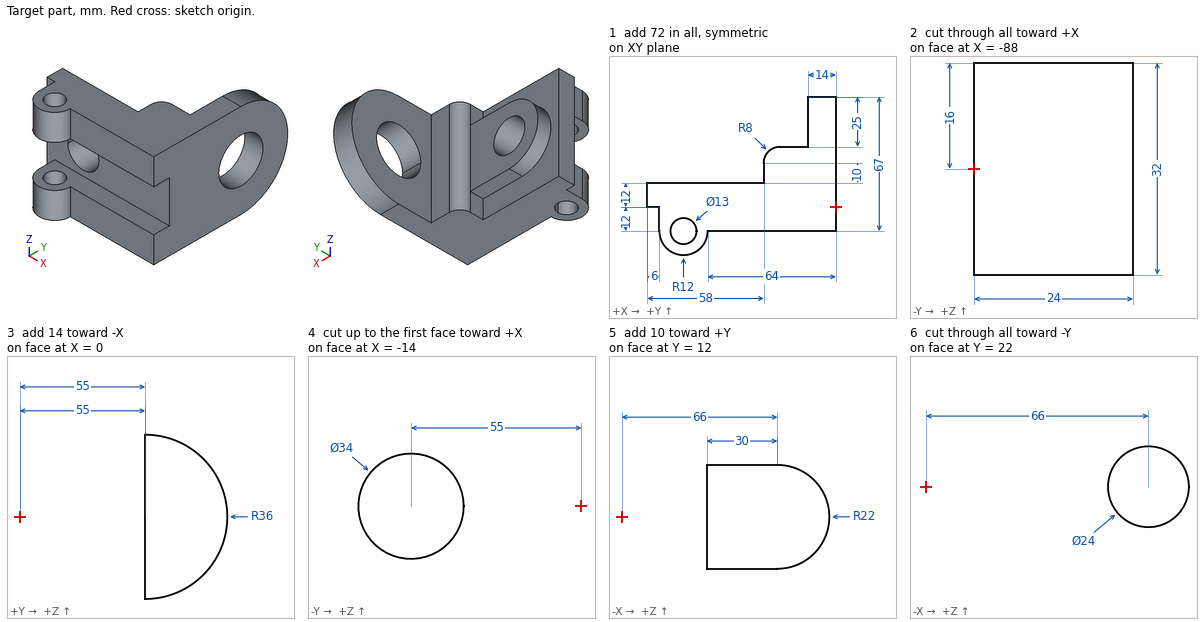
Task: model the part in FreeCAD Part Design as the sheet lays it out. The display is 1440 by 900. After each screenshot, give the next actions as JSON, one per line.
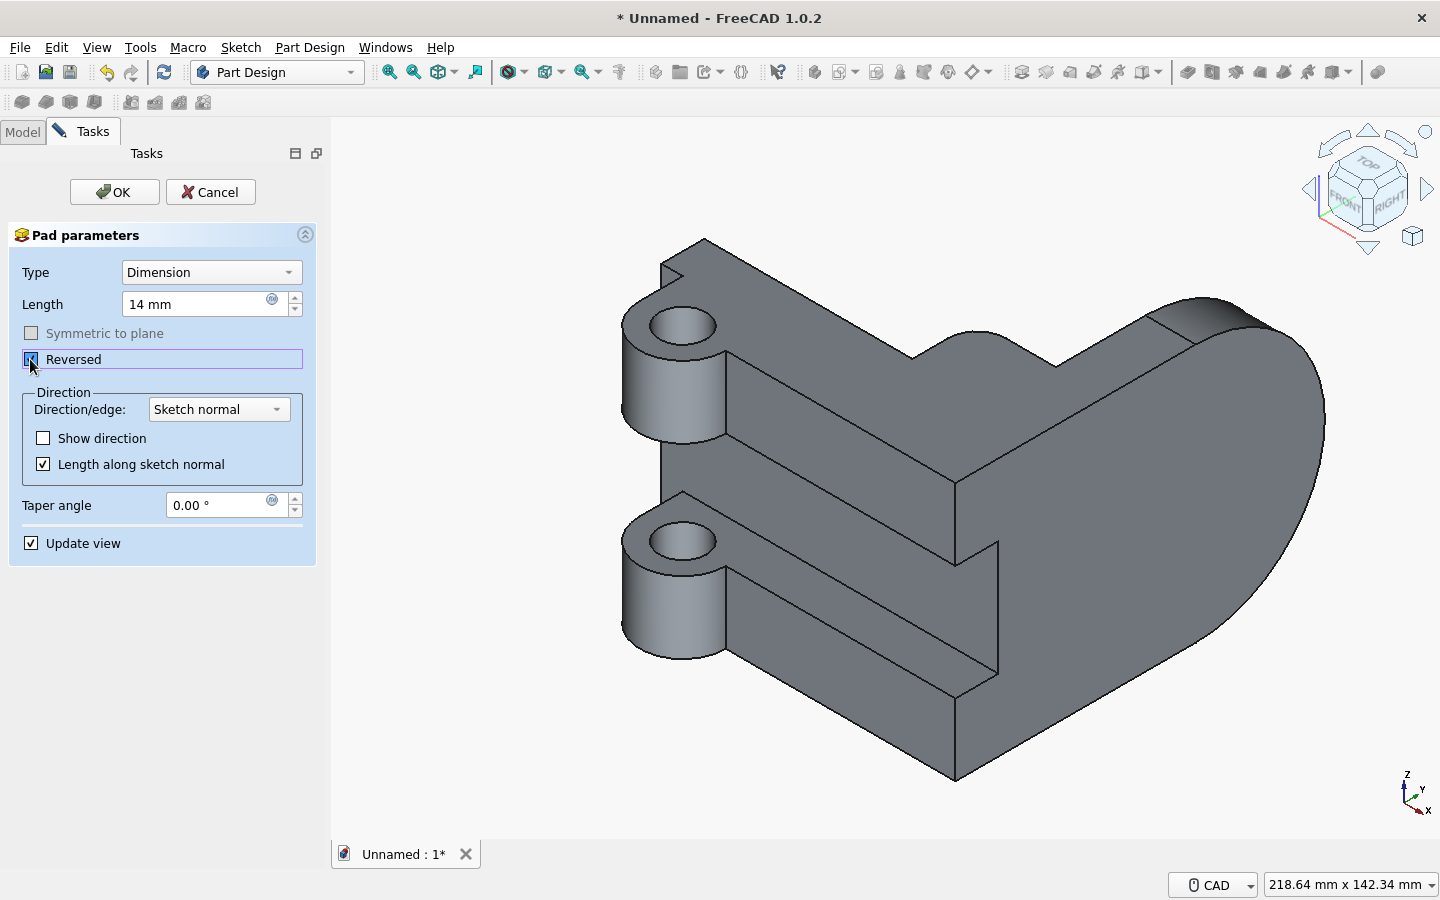
{"action": "left_click", "coordinate": [115, 192]}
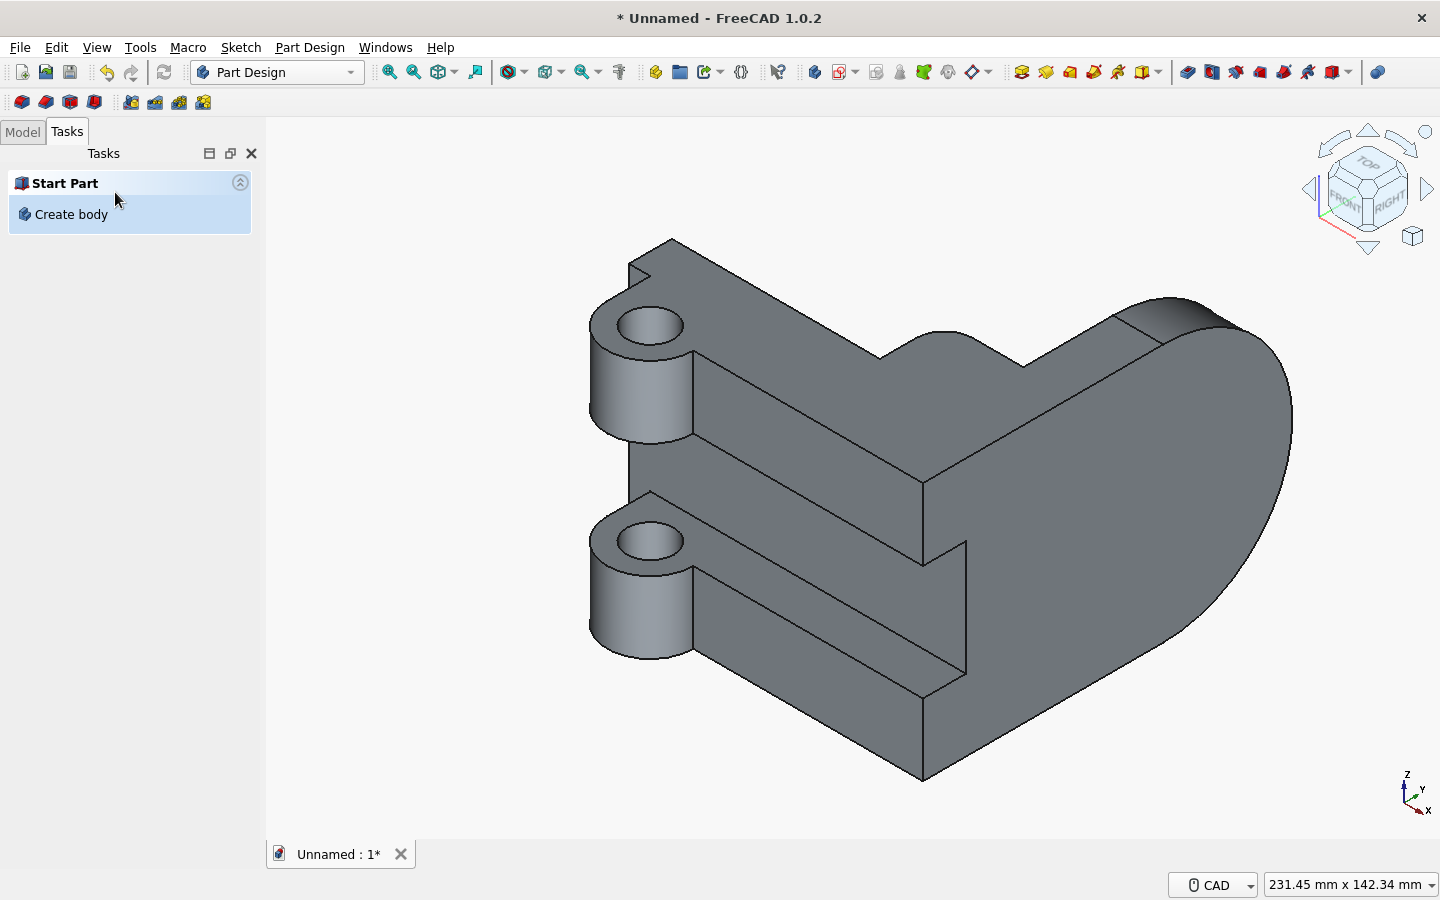
{"action": "left_click", "coordinate": [390, 72]}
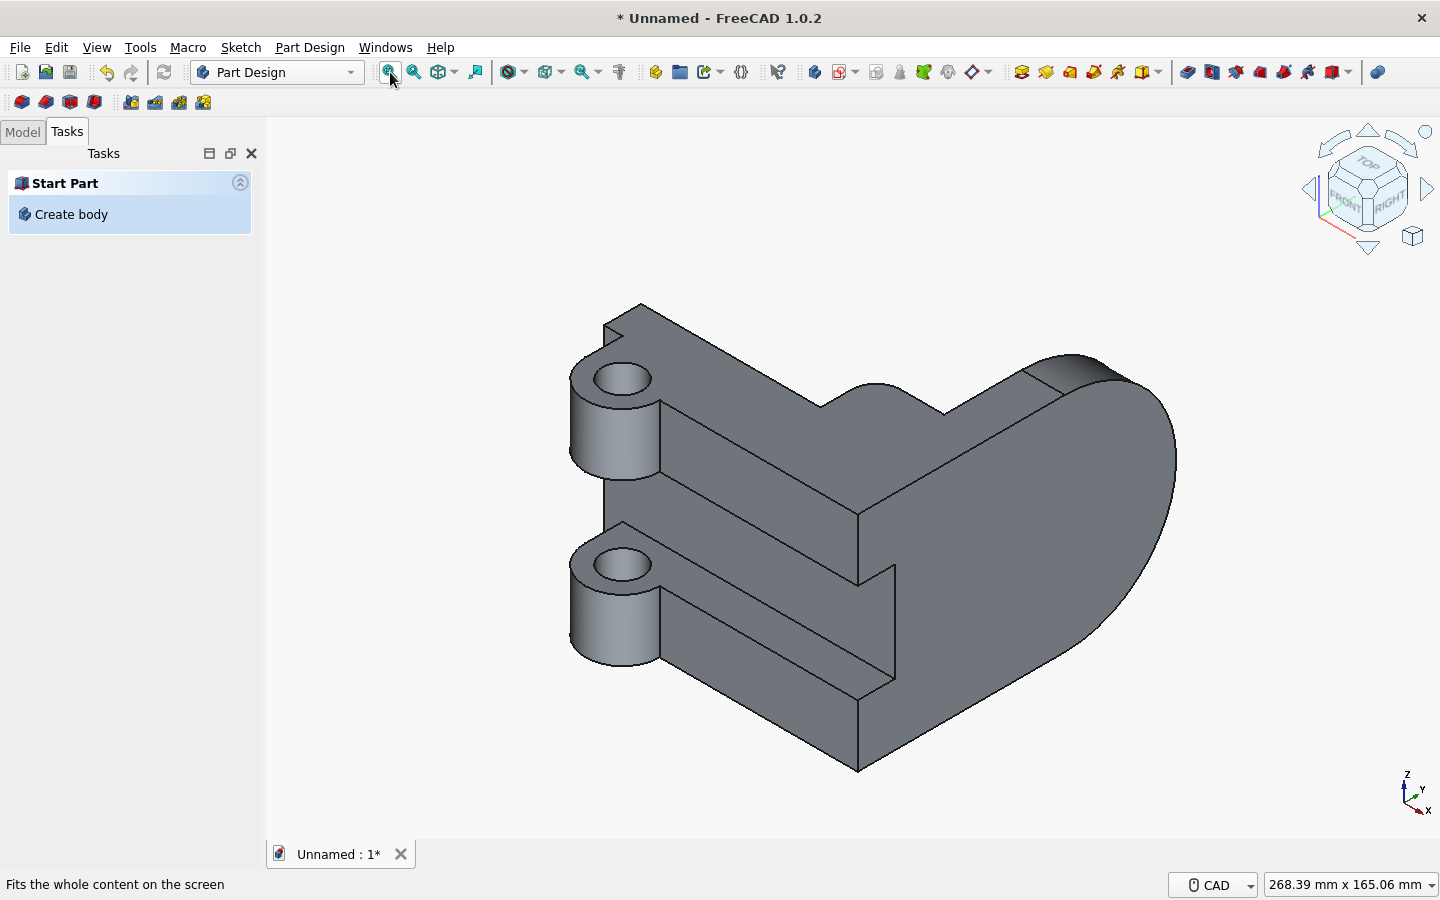
{"action": "key", "text": "6"}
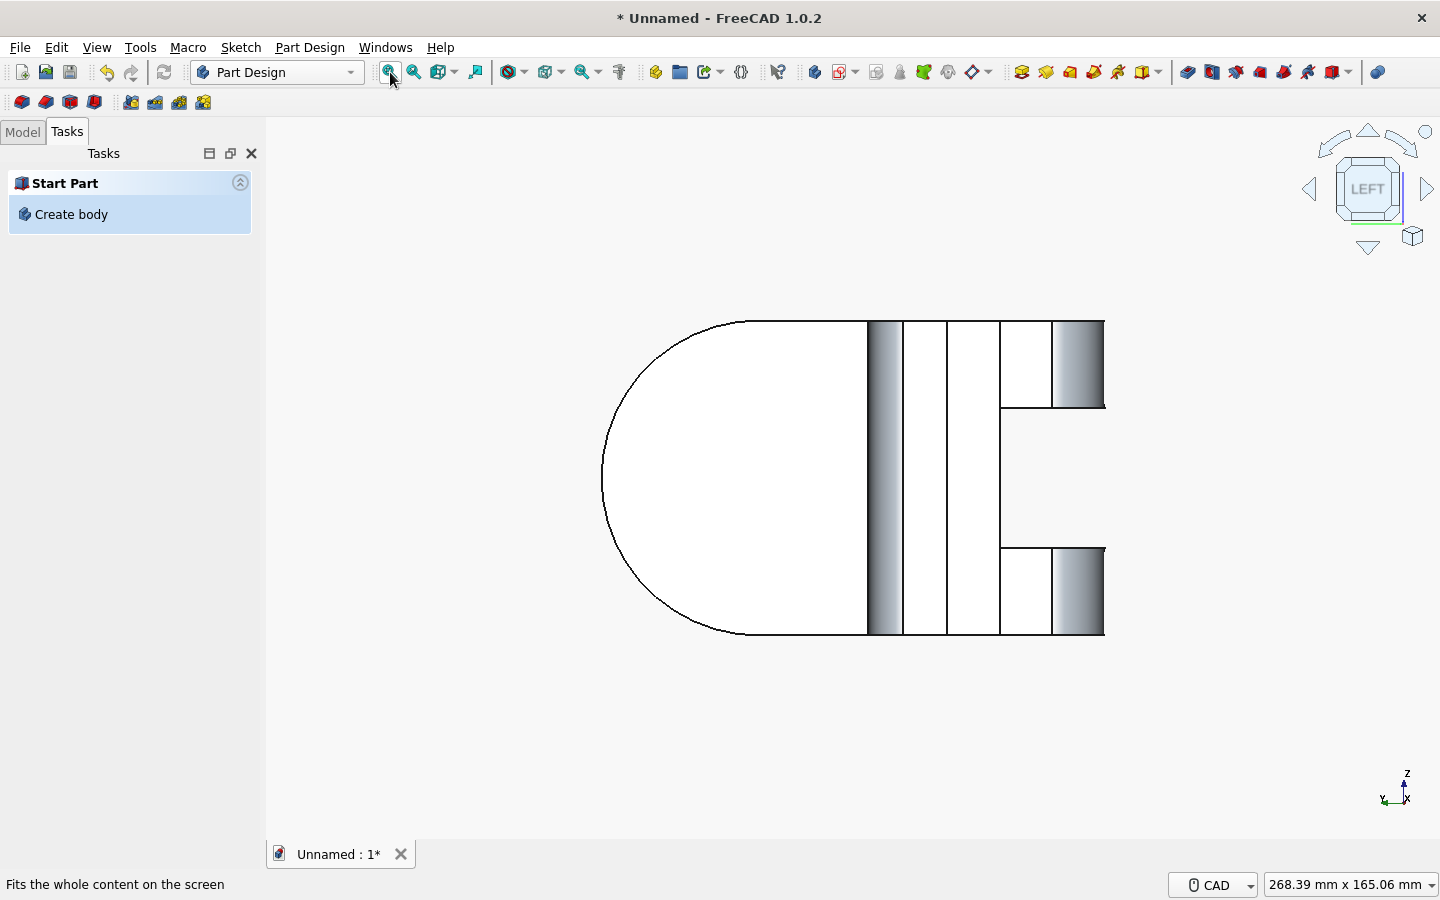
{"action": "left_click", "coordinate": [390, 72]}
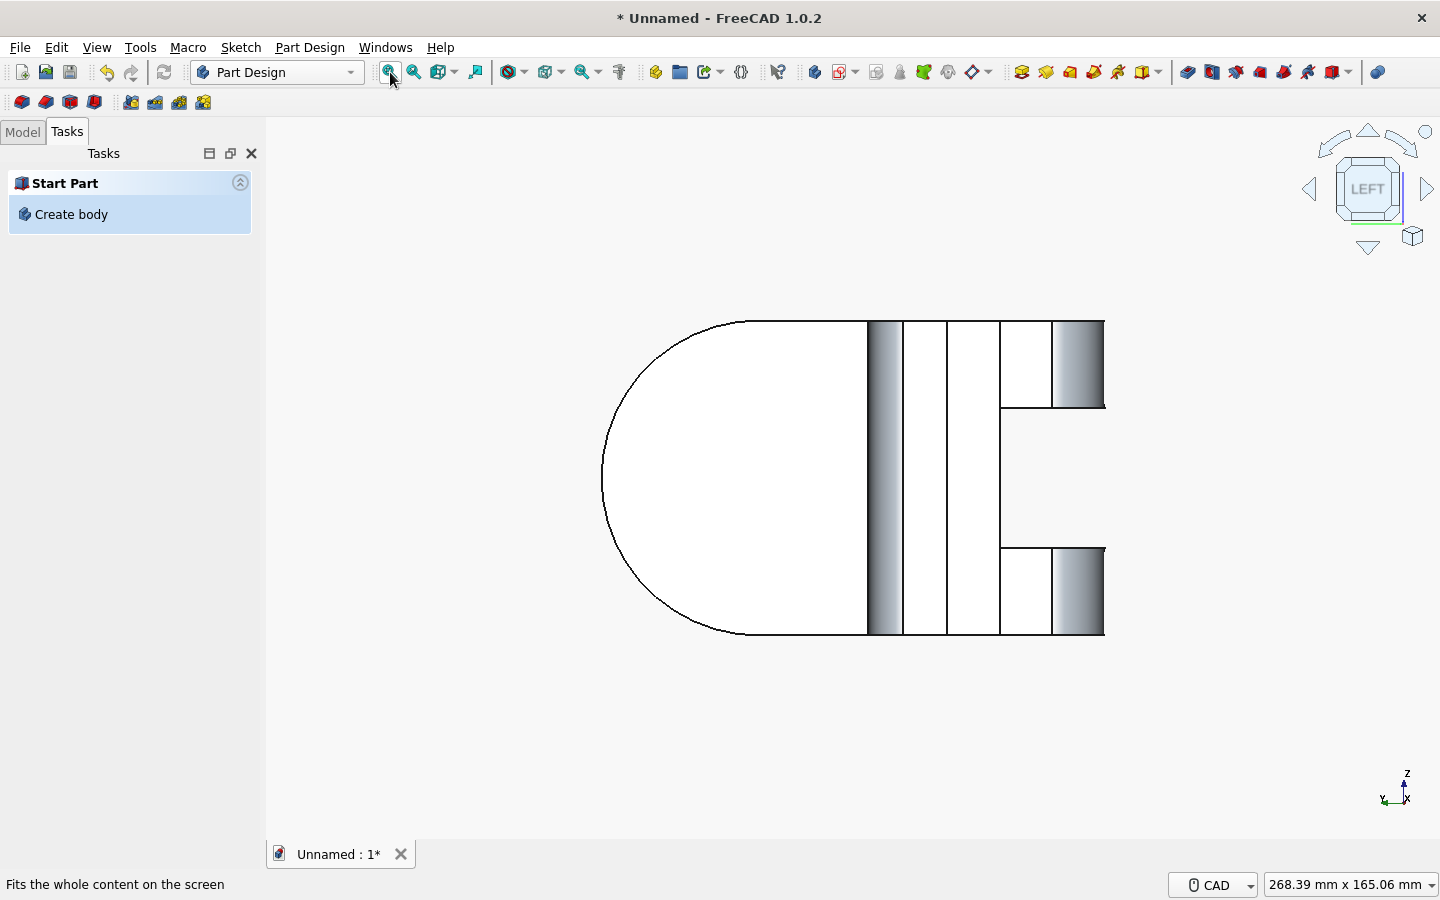
{"action": "left_click", "coordinate": [735, 477]}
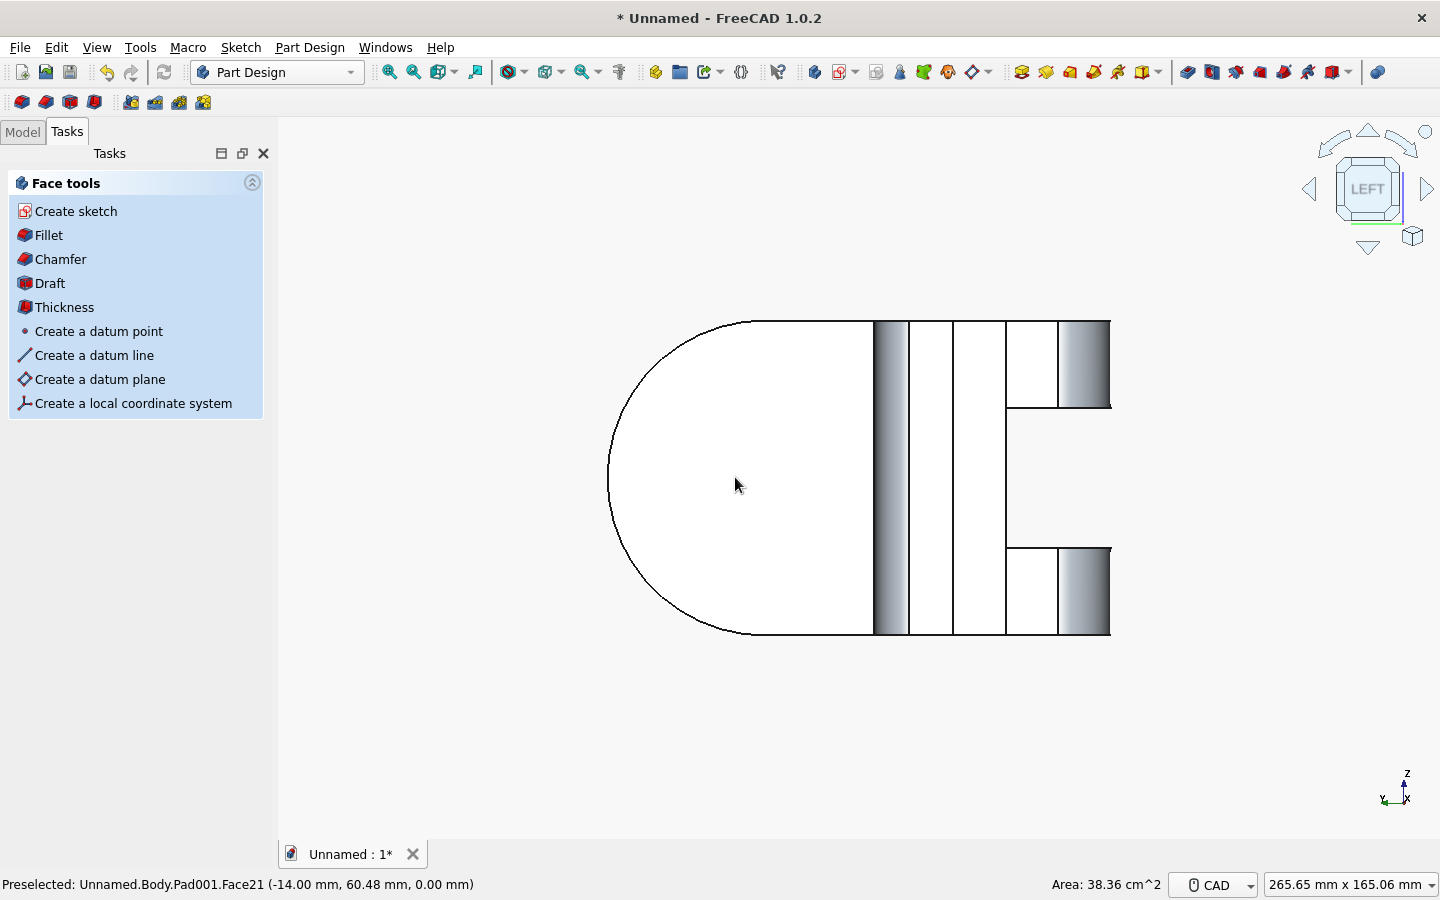
{"action": "left_click", "coordinate": [840, 72]}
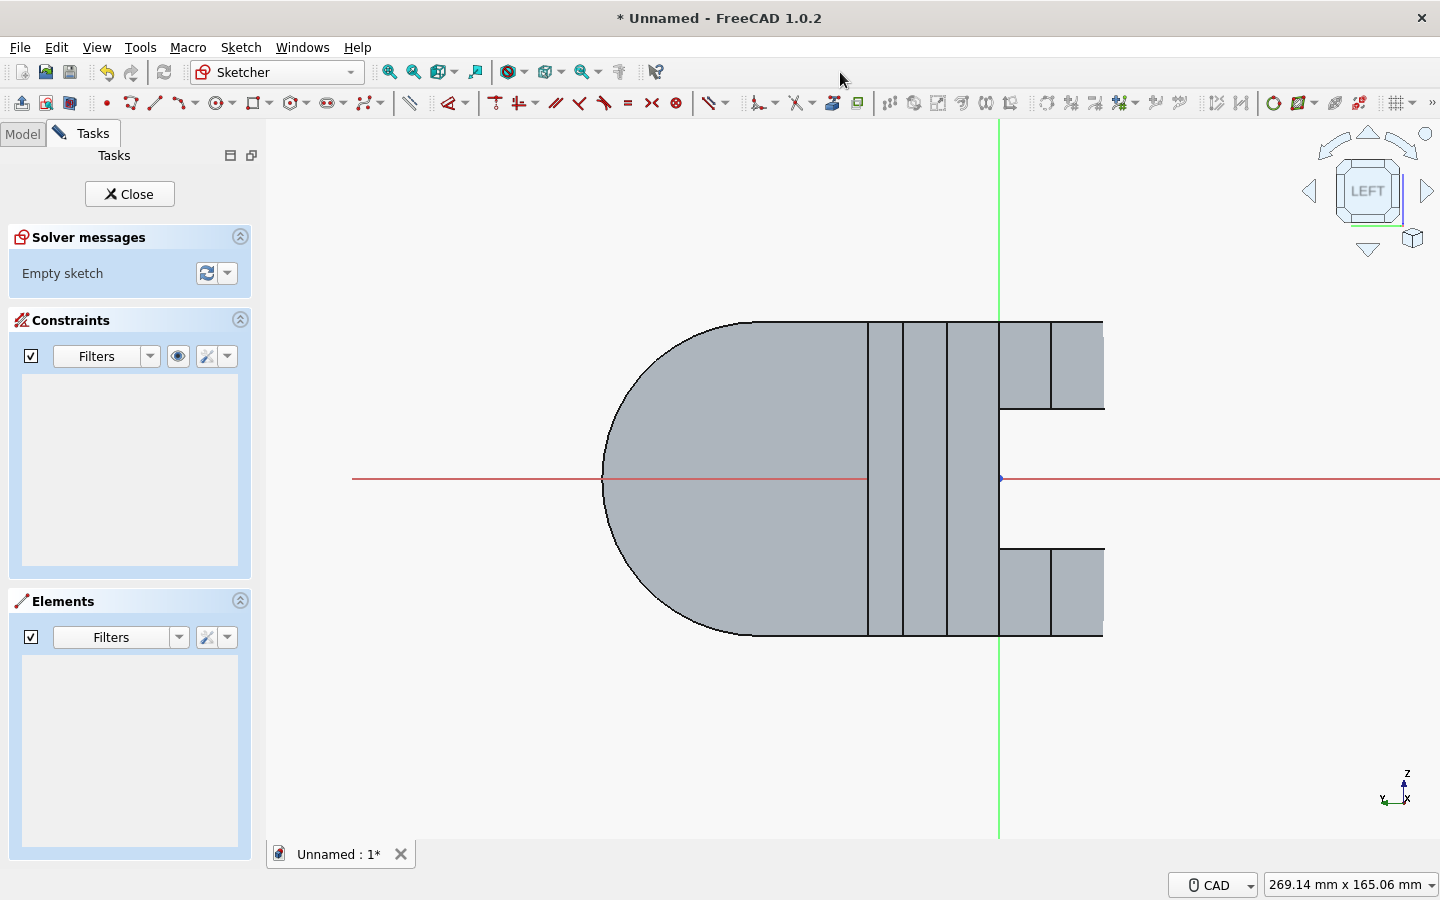
{"action": "left_click", "coordinate": [70, 104]}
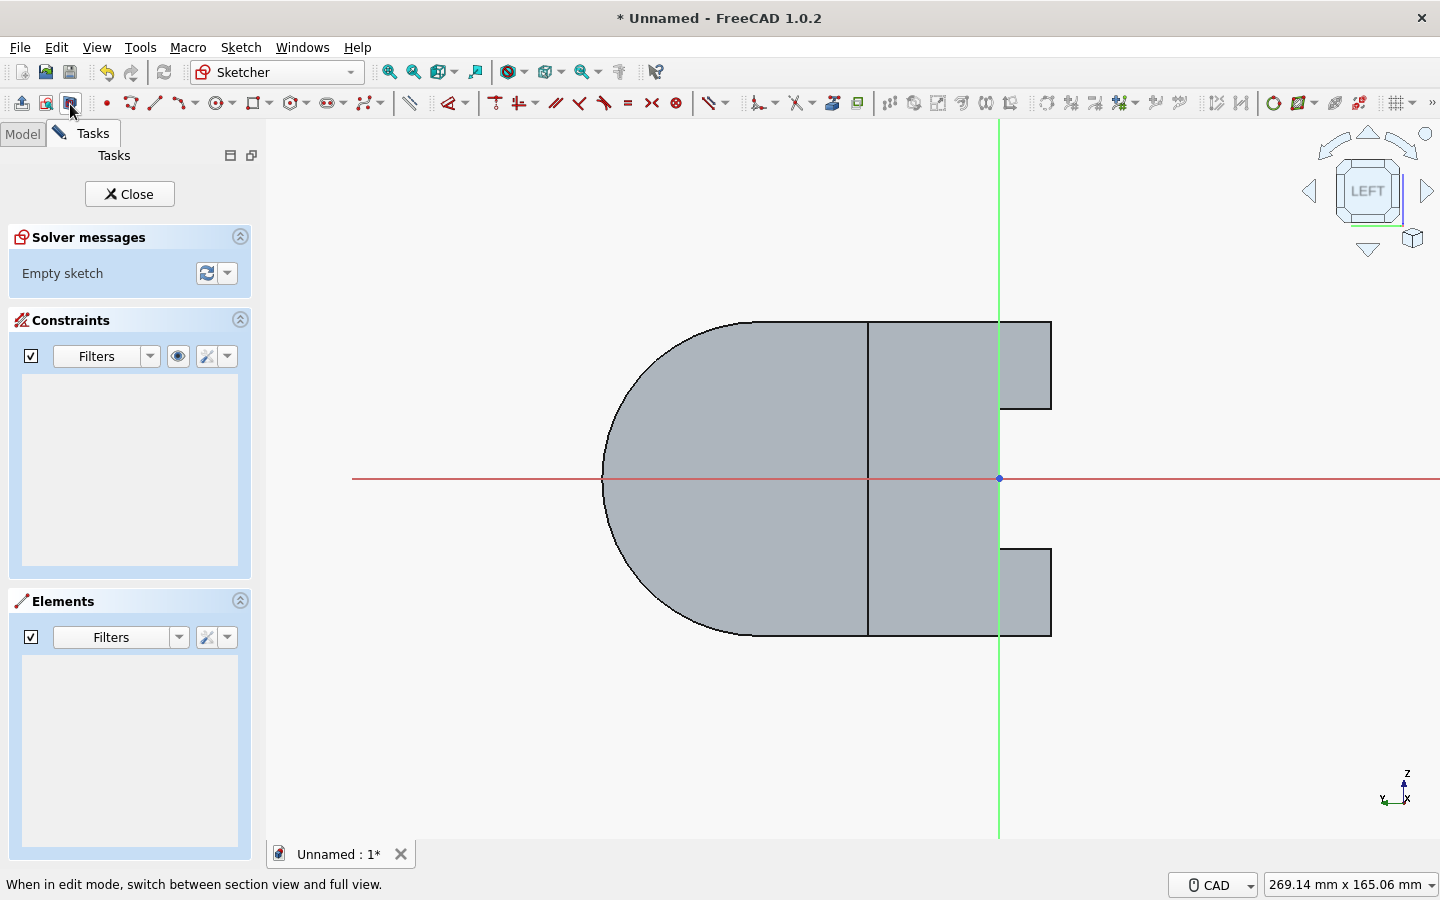
{"action": "scroll", "coordinate": [889, 479], "scroll_direction": "up", "scroll_amount": 4}